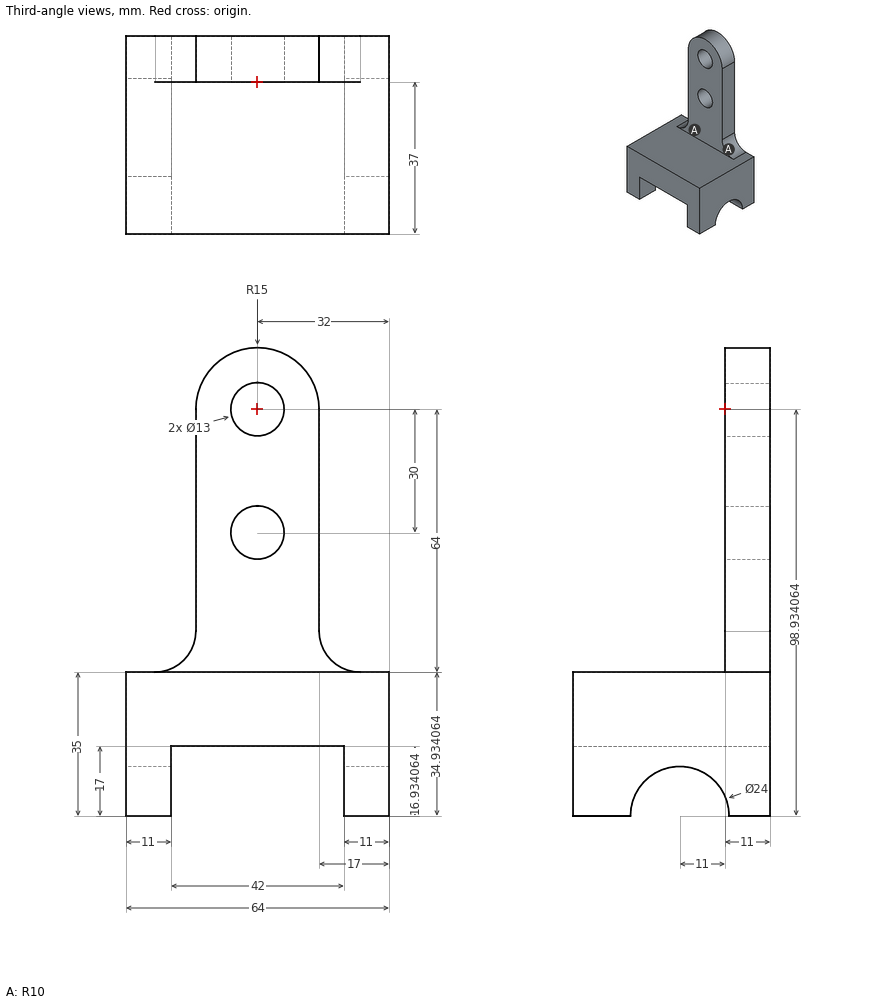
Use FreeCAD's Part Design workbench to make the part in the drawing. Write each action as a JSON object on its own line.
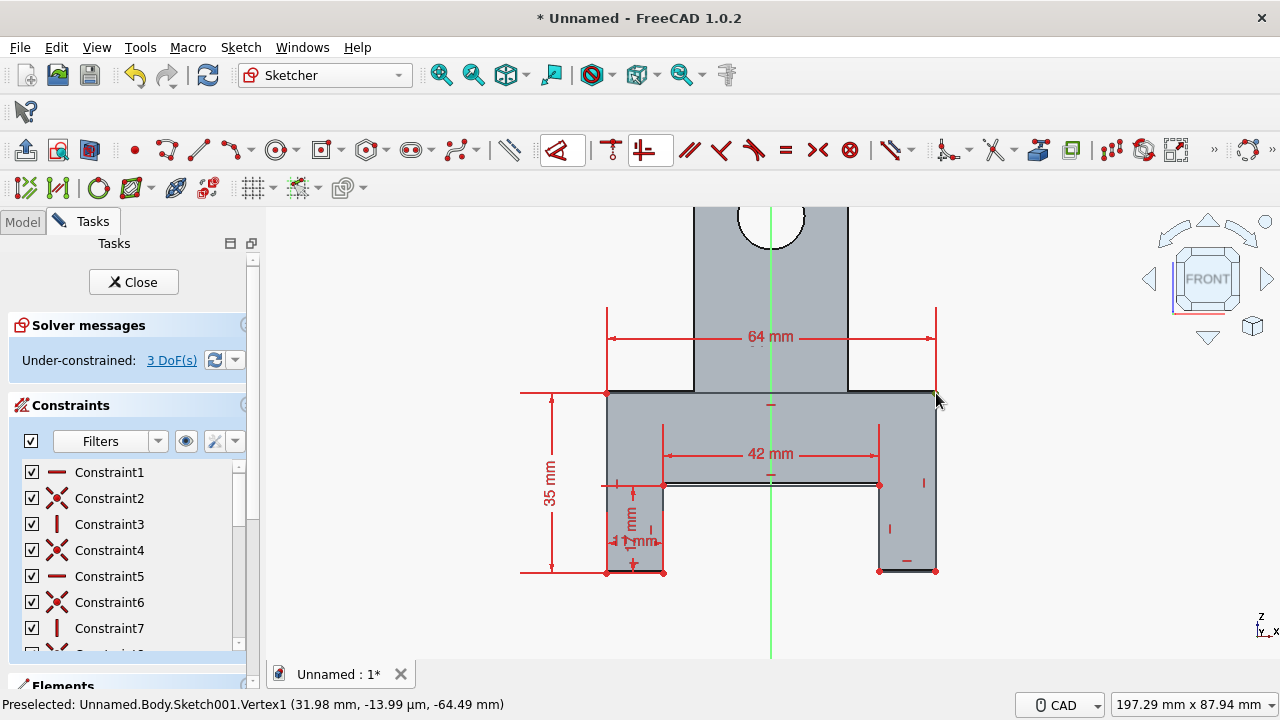
{"action": "key", "text": "l"}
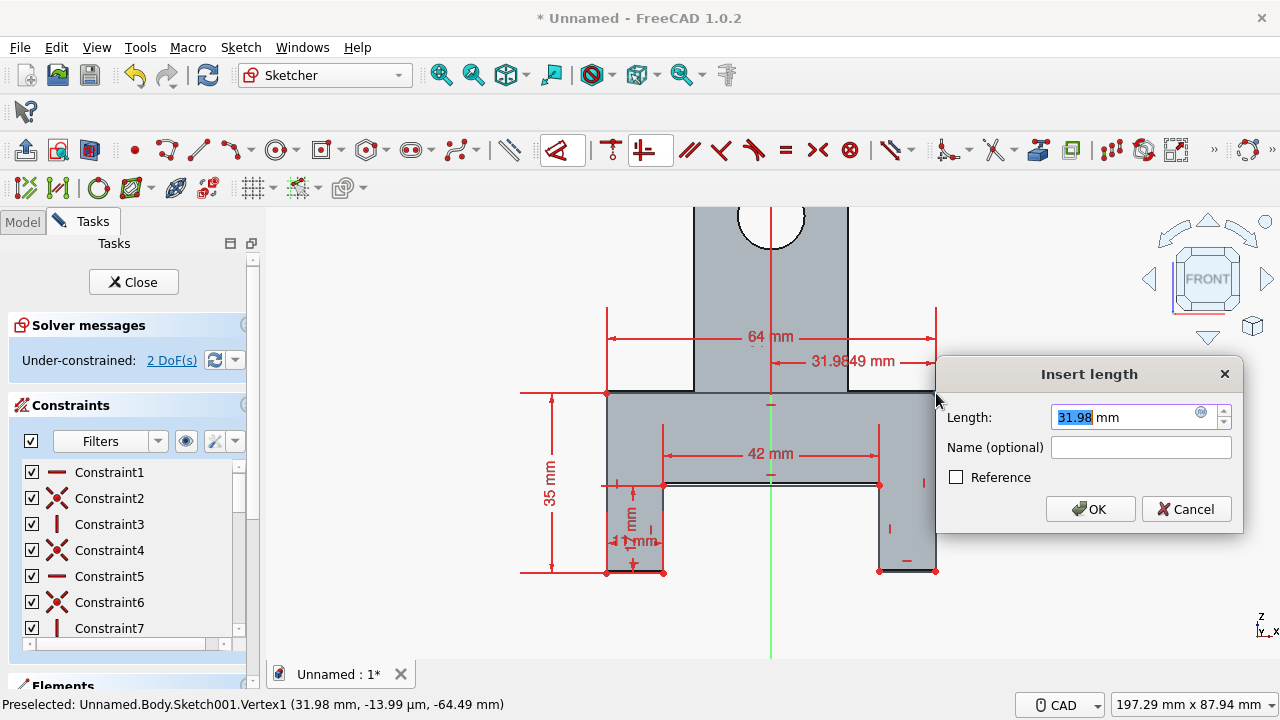
{"action": "type", "text": "32"}
{"action": "key", "text": "Return"}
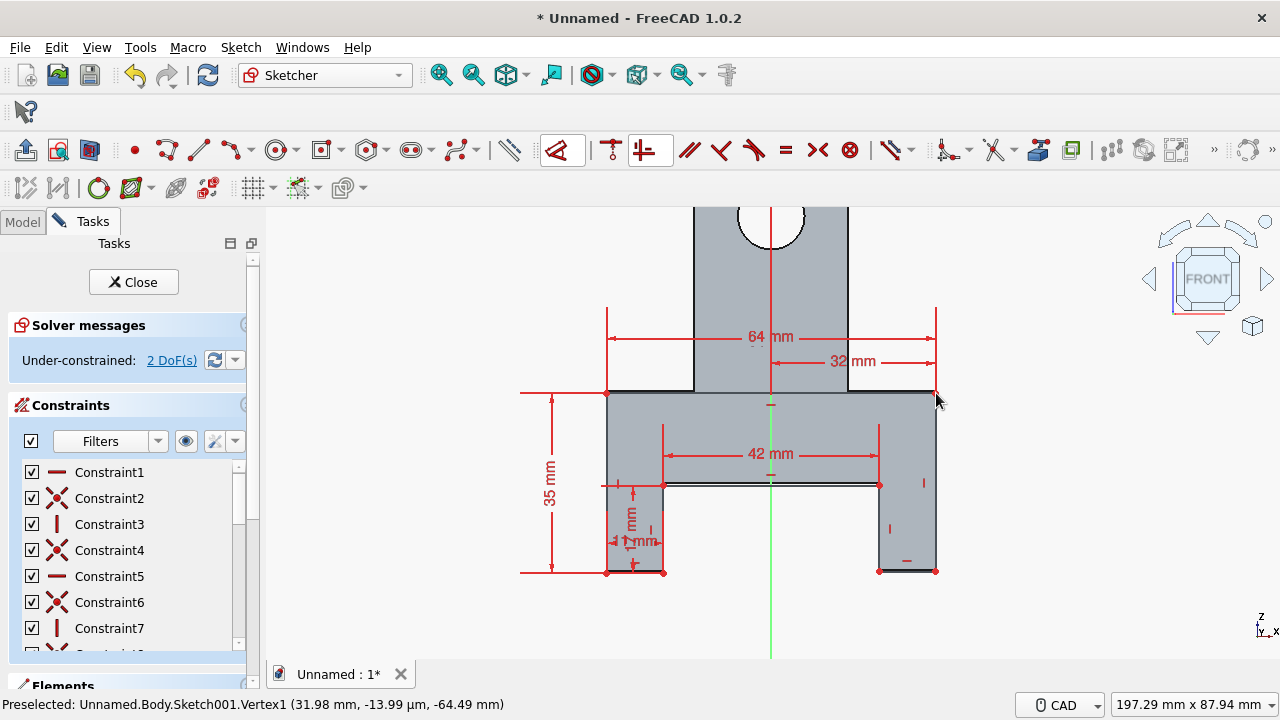
{"action": "left_click", "coordinate": [936, 393]}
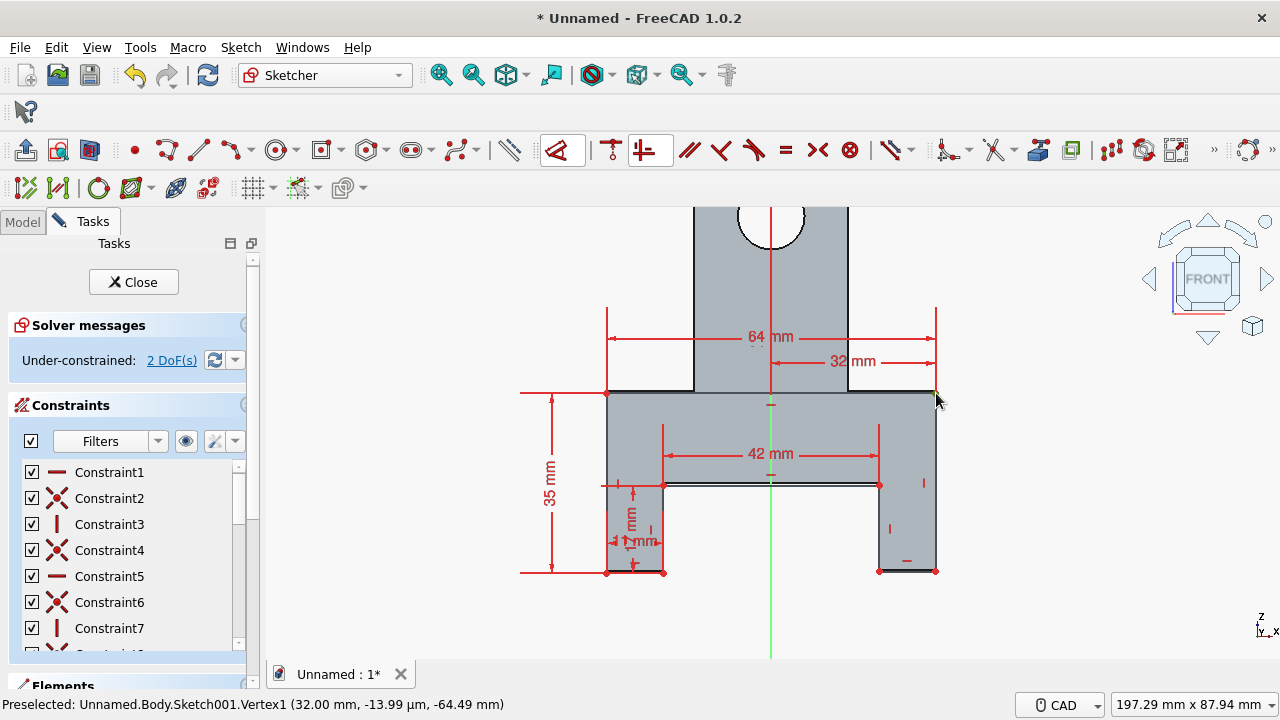
{"action": "left_click", "coordinate": [580, 150]}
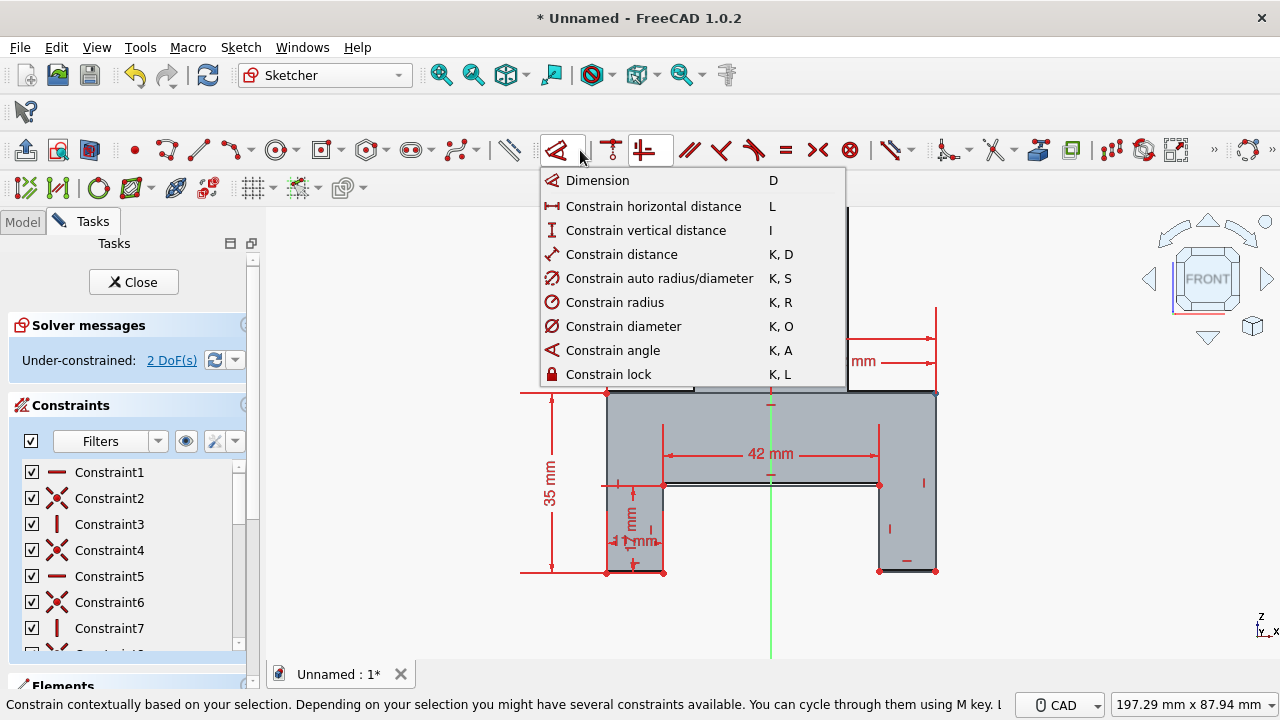
{"action": "left_click", "coordinate": [693, 230]}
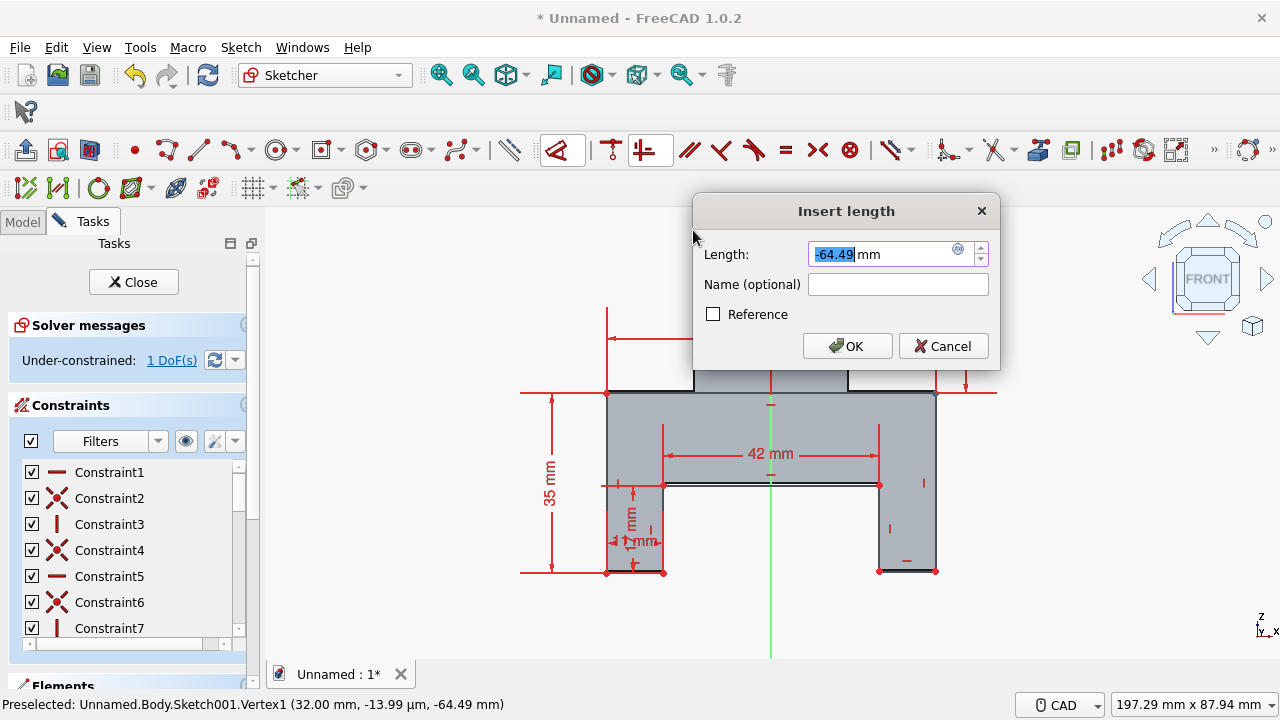
{"action": "type", "text": "-64"}
{"action": "key", "text": "Return"}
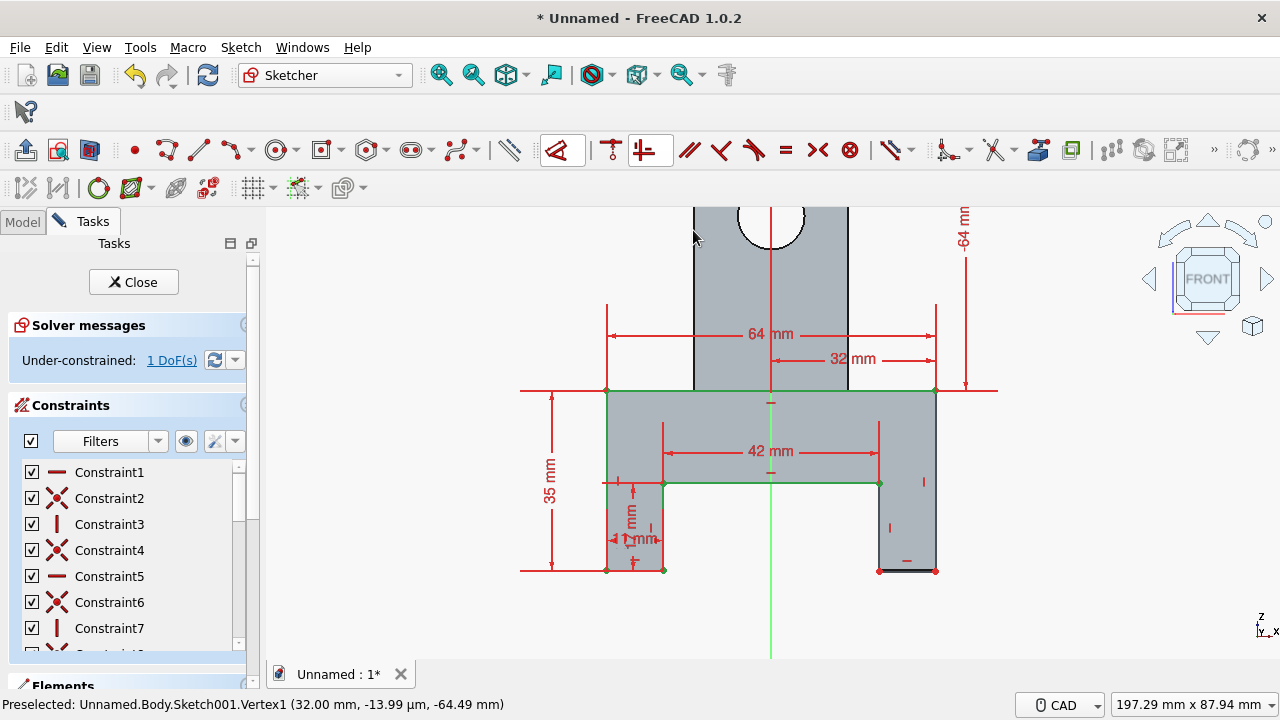
{"action": "left_click", "coordinate": [879, 510]}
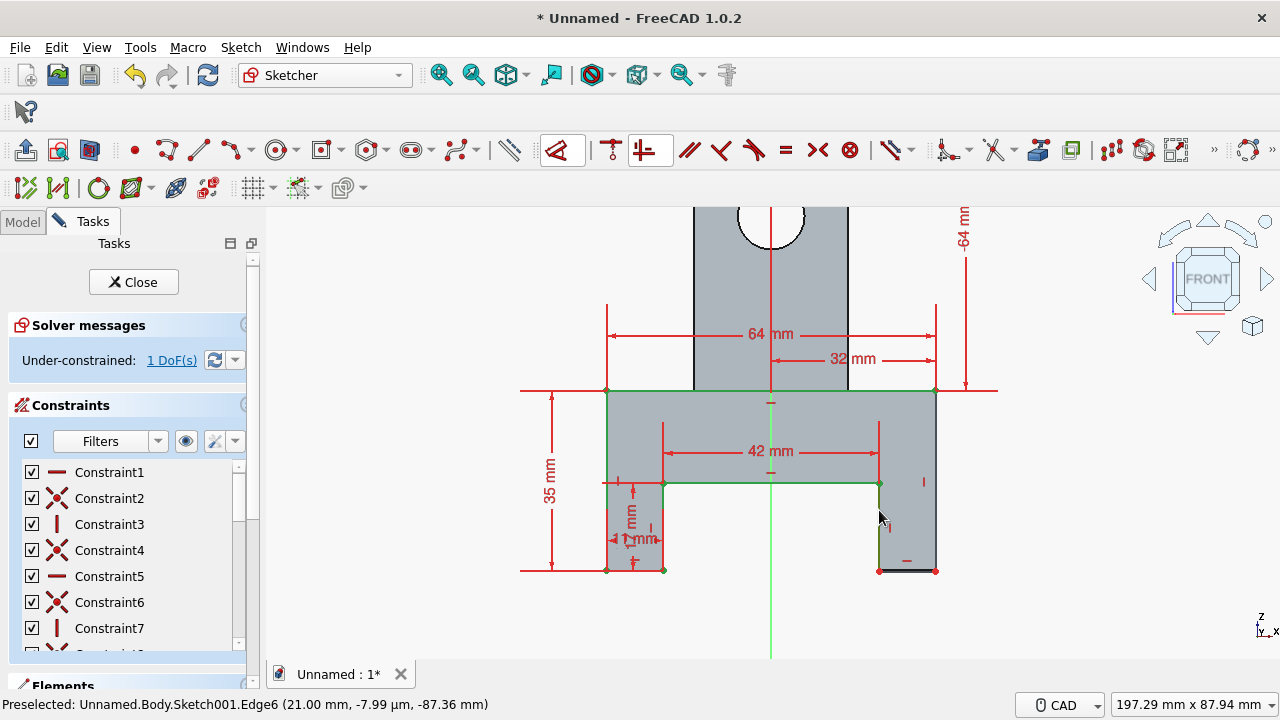
{"action": "left_click", "coordinate": [580, 150]}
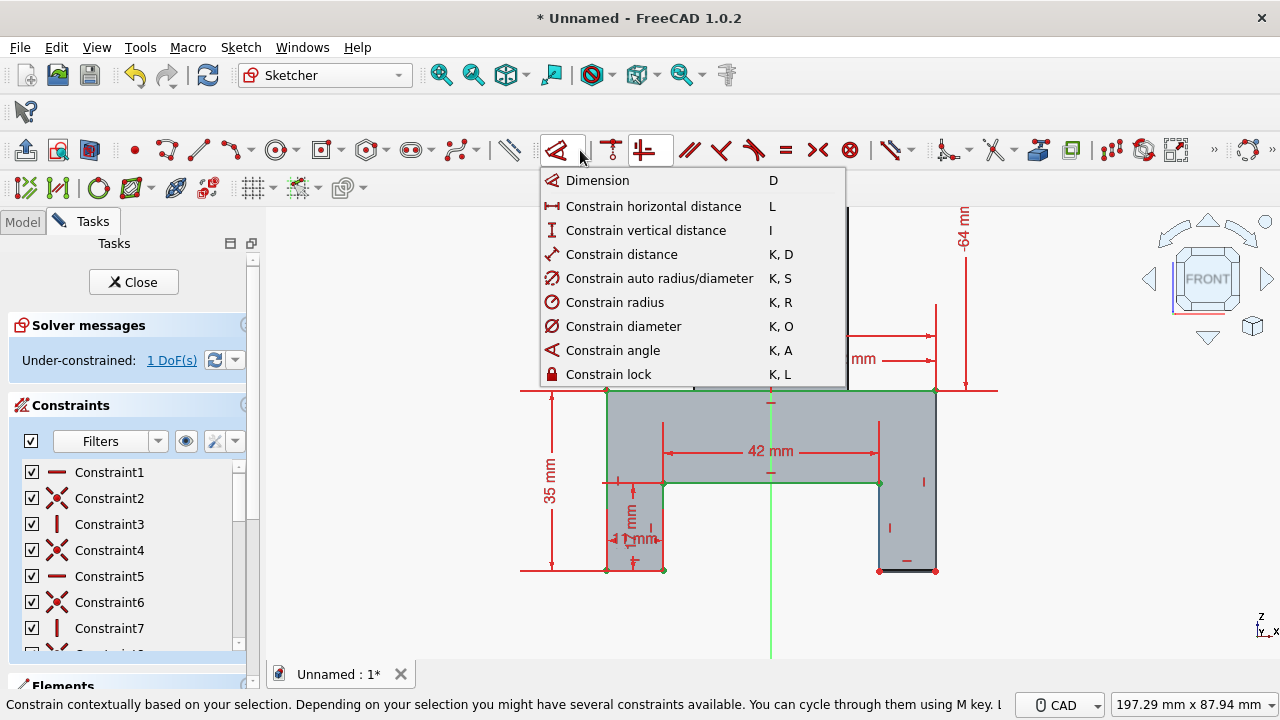
{"action": "left_click", "coordinate": [693, 230]}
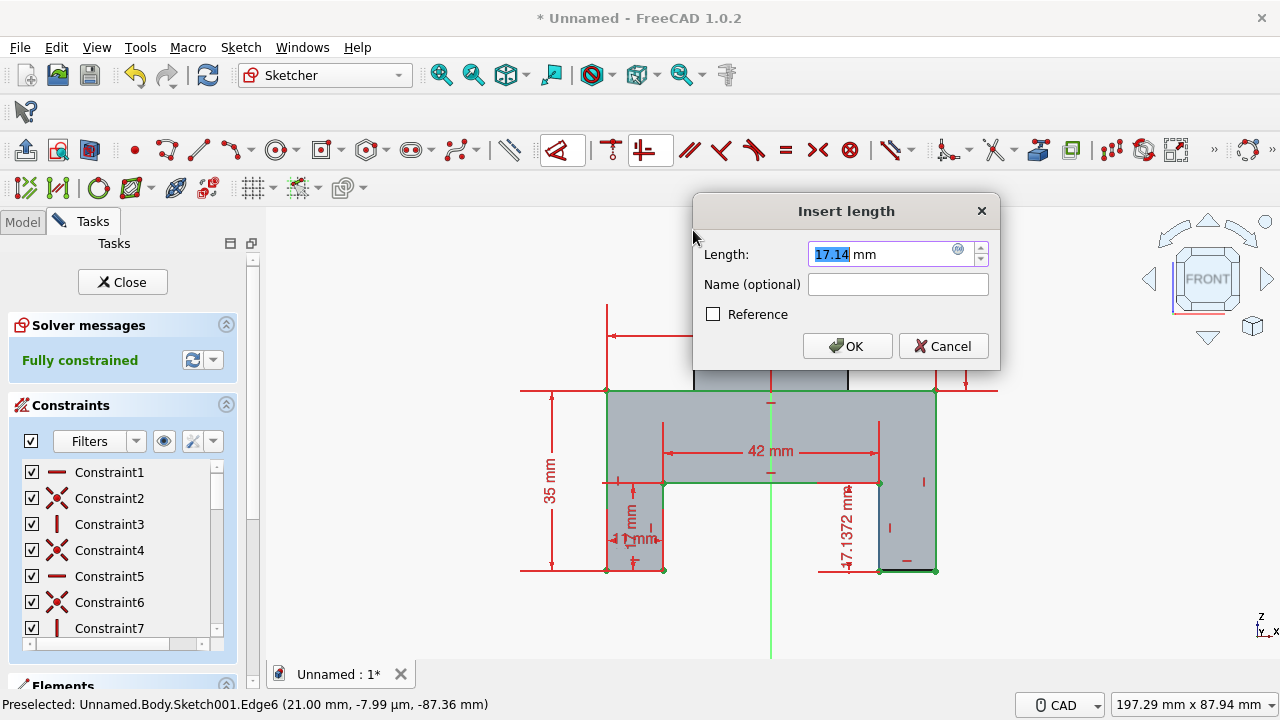
{"action": "type", "text": "16.934064"}
{"action": "key", "text": "Return"}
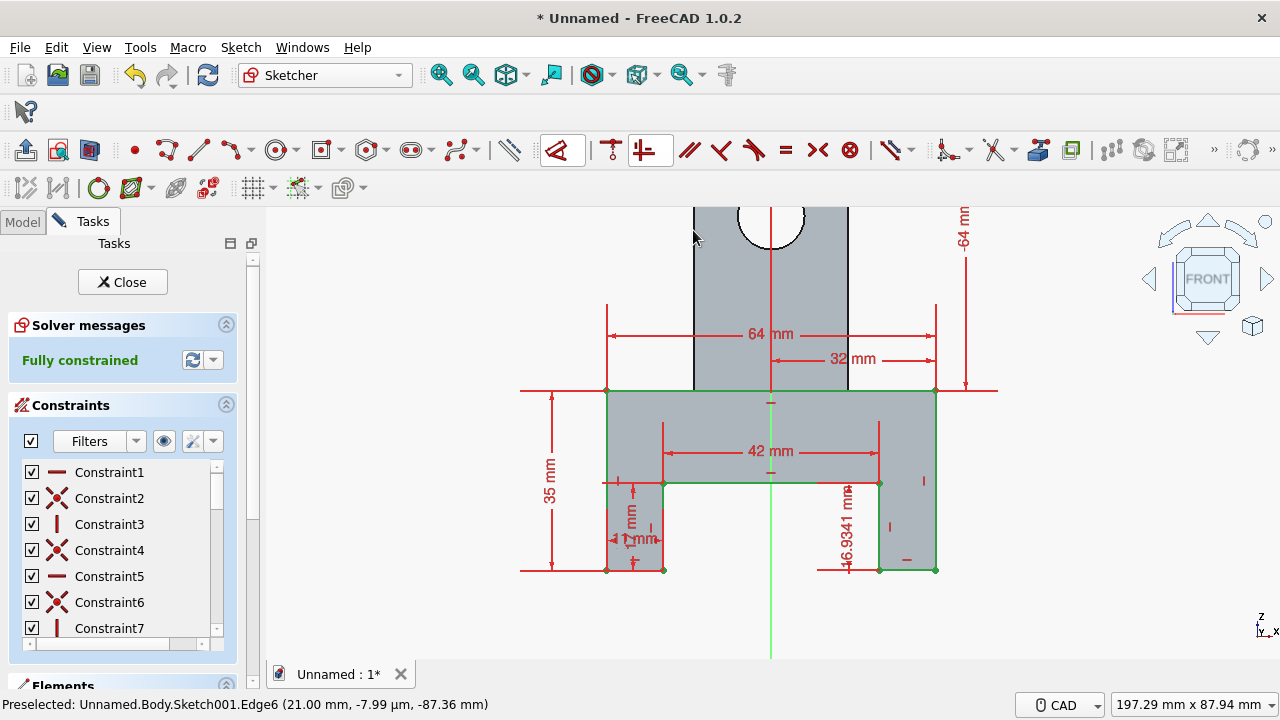
{"action": "left_click", "coordinate": [123, 282]}